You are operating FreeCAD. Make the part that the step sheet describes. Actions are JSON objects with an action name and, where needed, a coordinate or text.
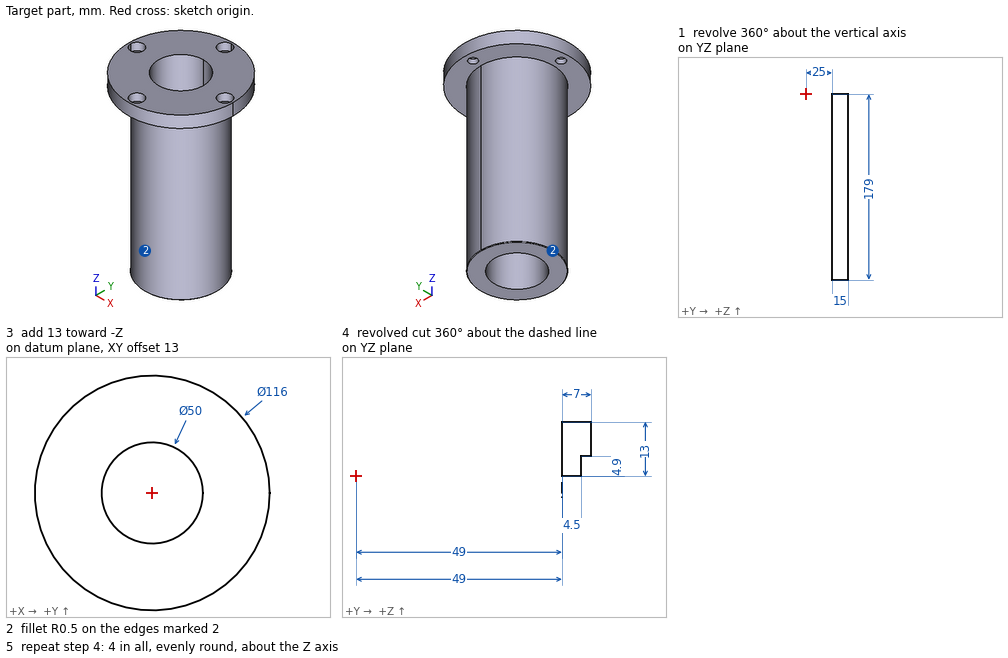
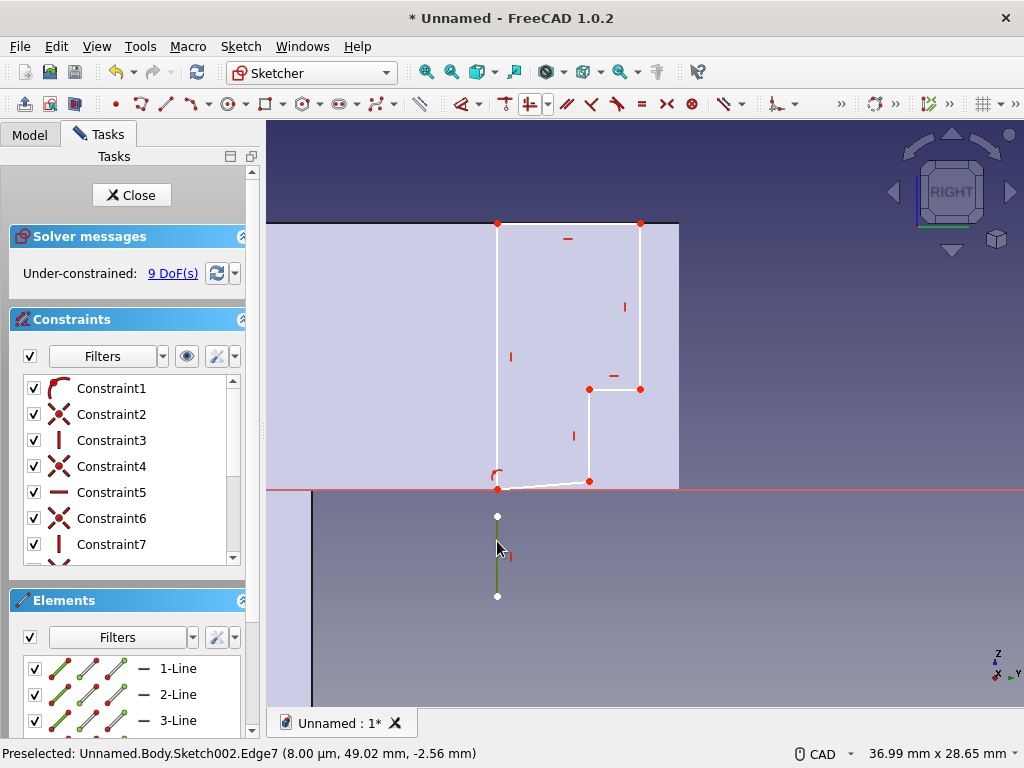
{"action": "left_click", "coordinate": [420, 104]}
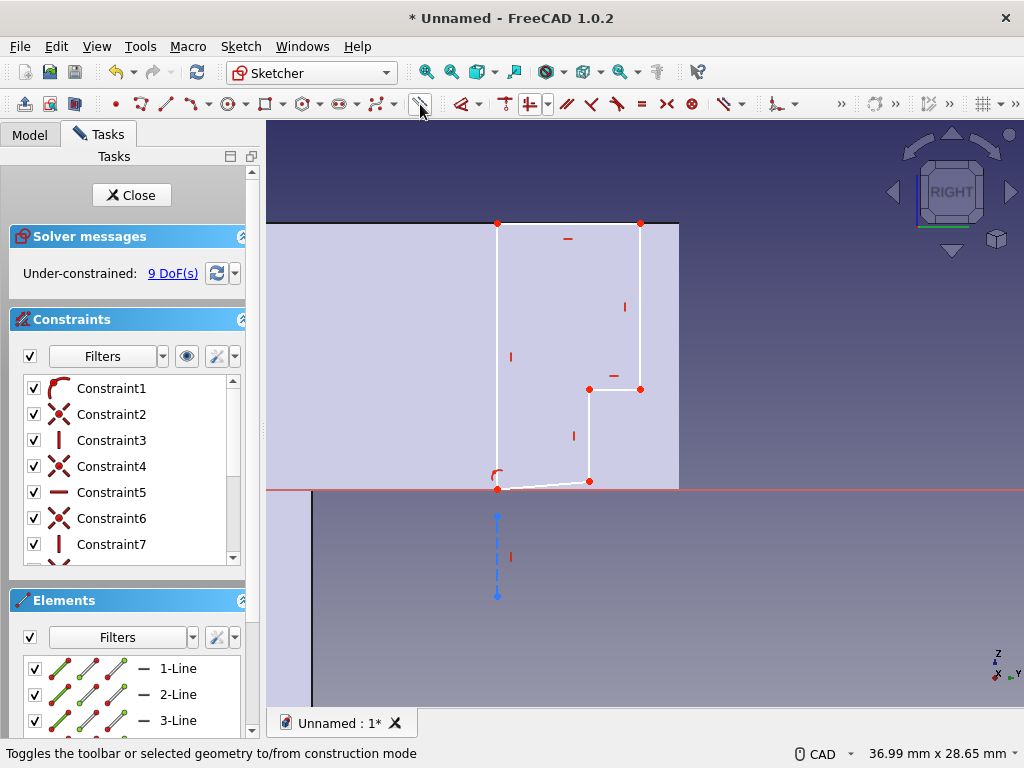
{"action": "left_click", "coordinate": [525, 487]}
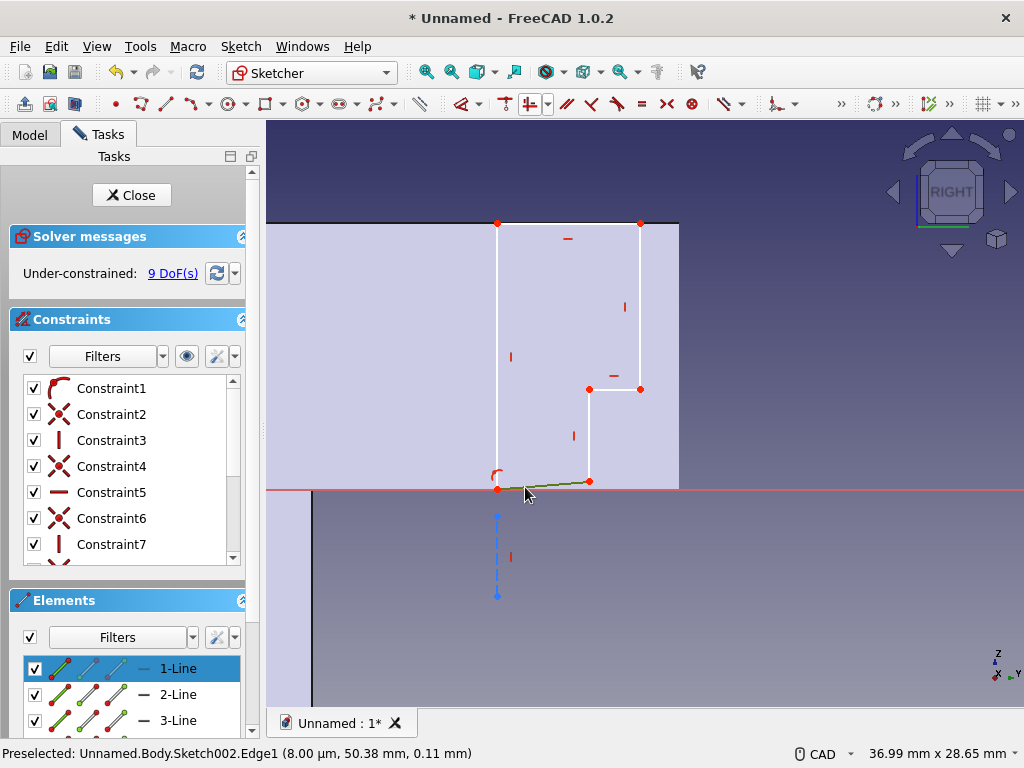
{"action": "left_click", "coordinate": [548, 104]}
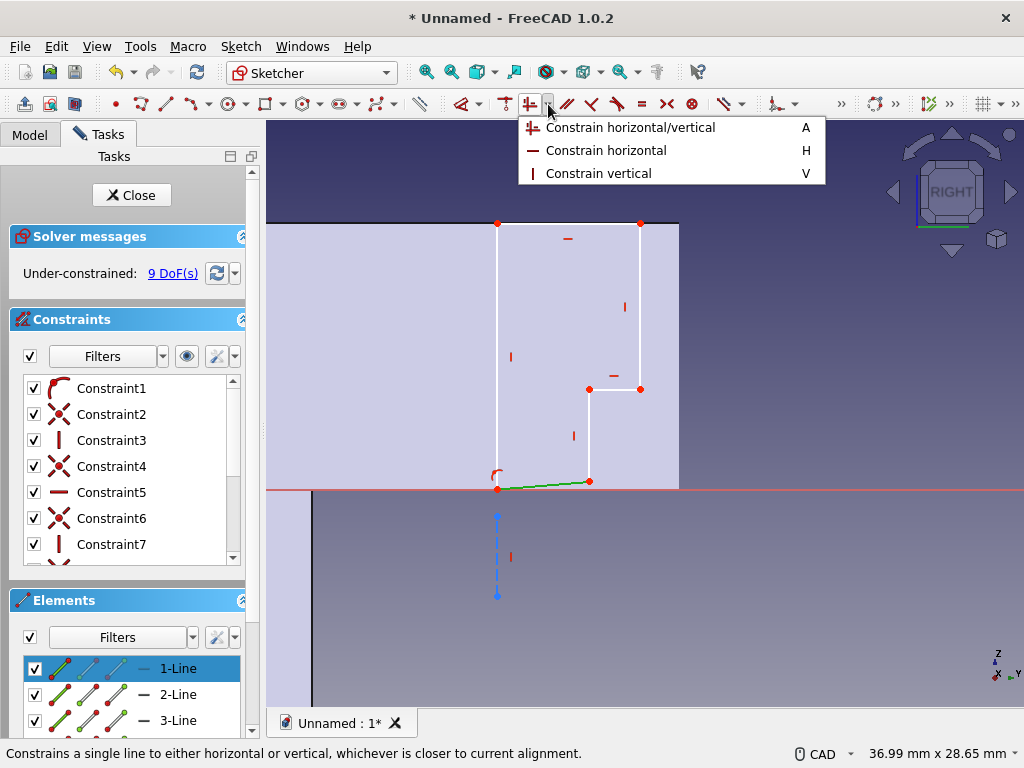
{"action": "left_click", "coordinate": [672, 150]}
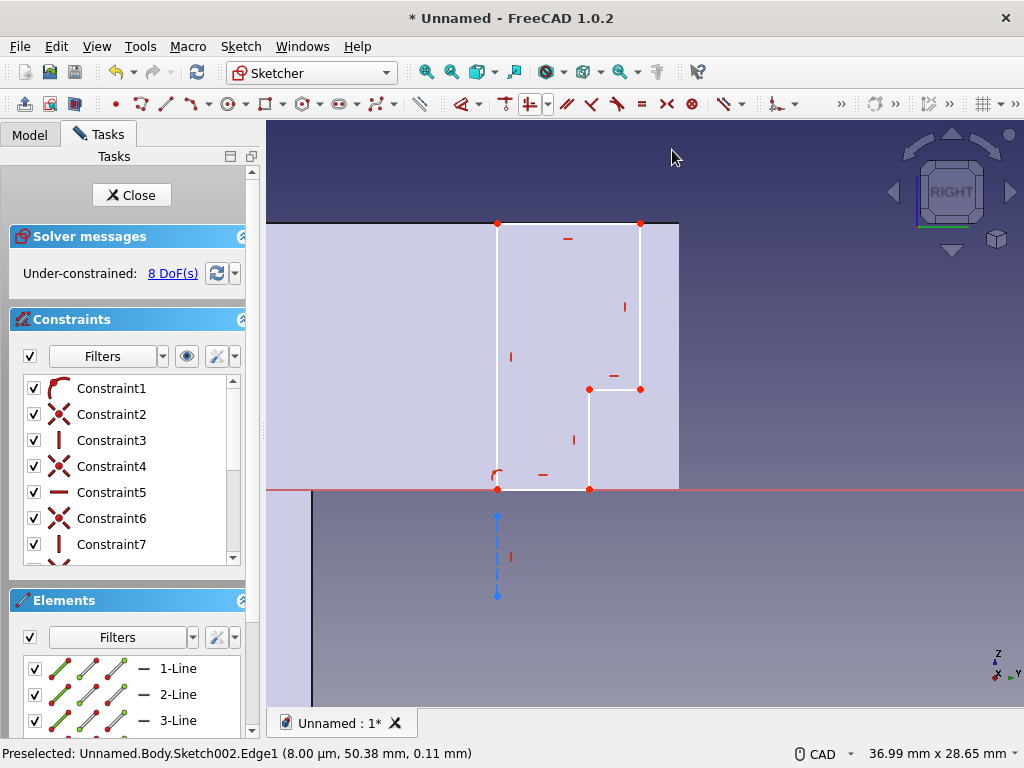
{"action": "left_click", "coordinate": [460, 104]}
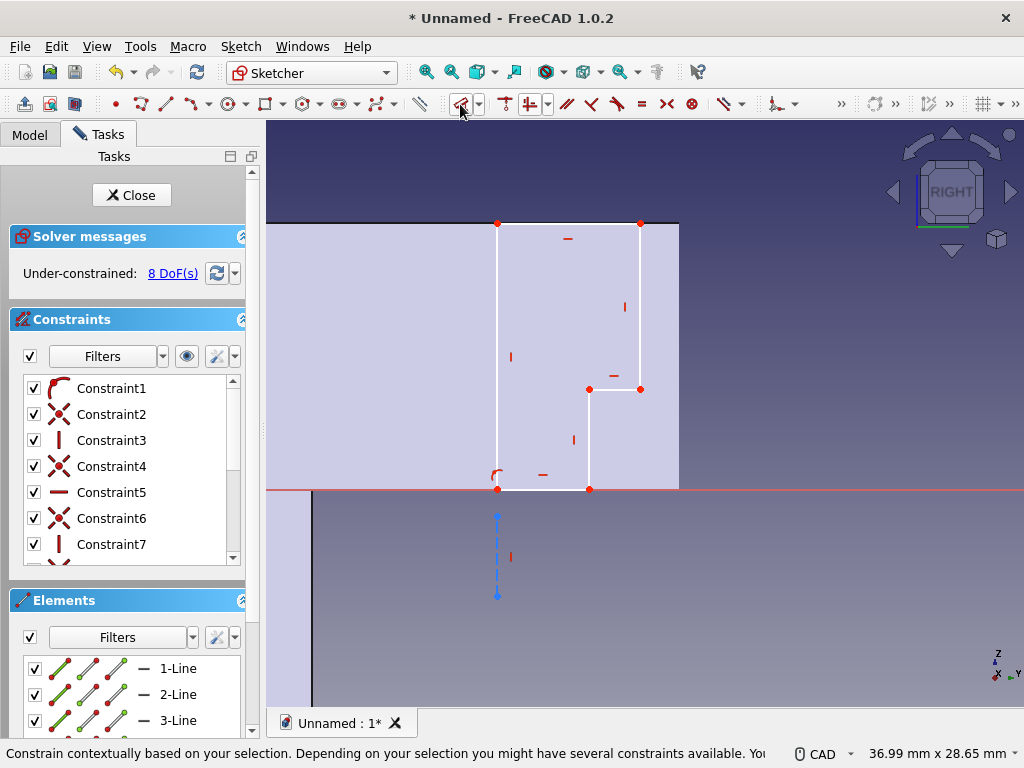
{"action": "left_click", "coordinate": [597, 224]}
{"action": "left_click", "coordinate": [568, 190]}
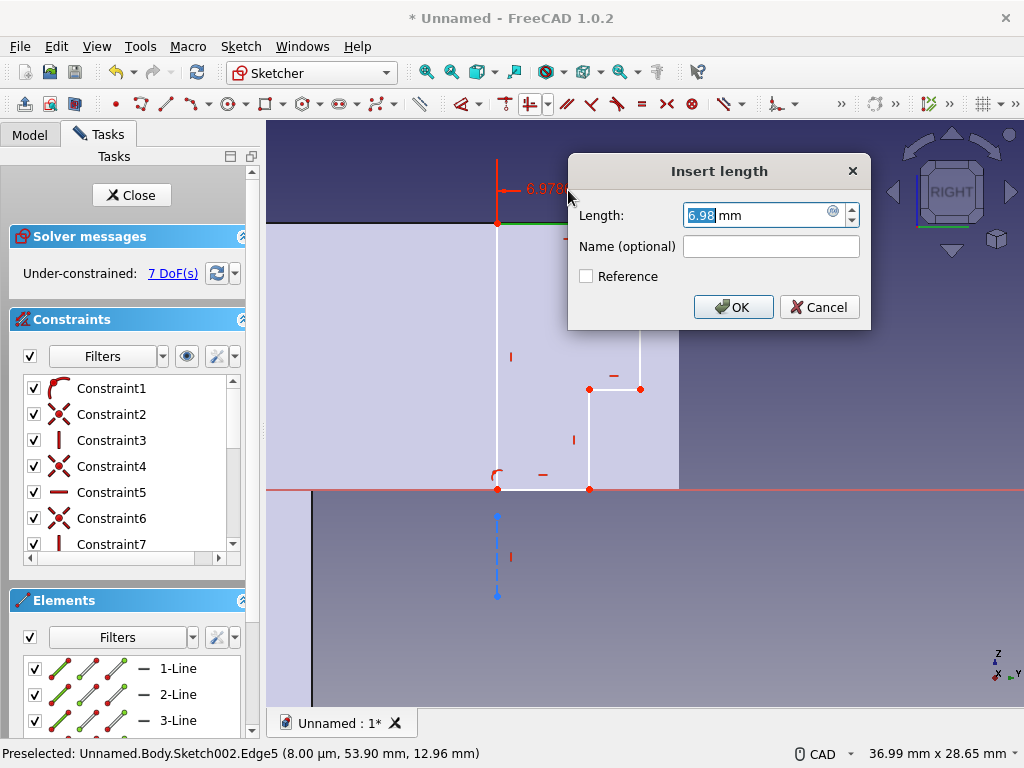
{"action": "type", "text": "7"}
{"action": "key", "text": "Return"}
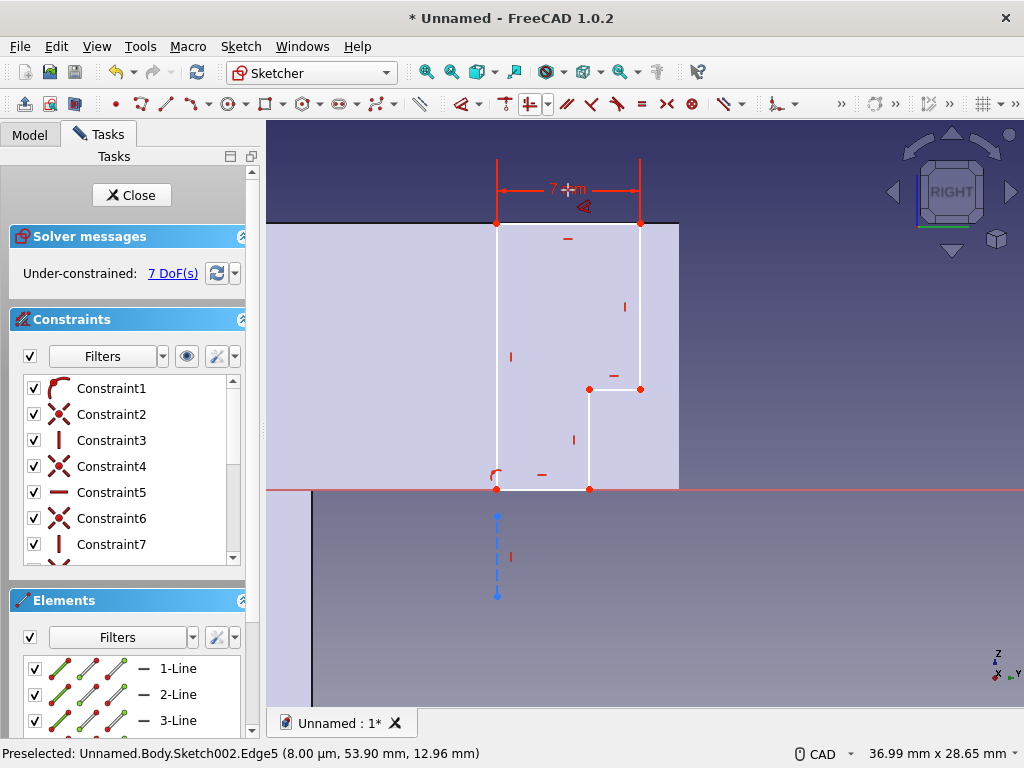
{"action": "left_click", "coordinate": [497, 304]}
{"action": "left_click", "coordinate": [463, 357]}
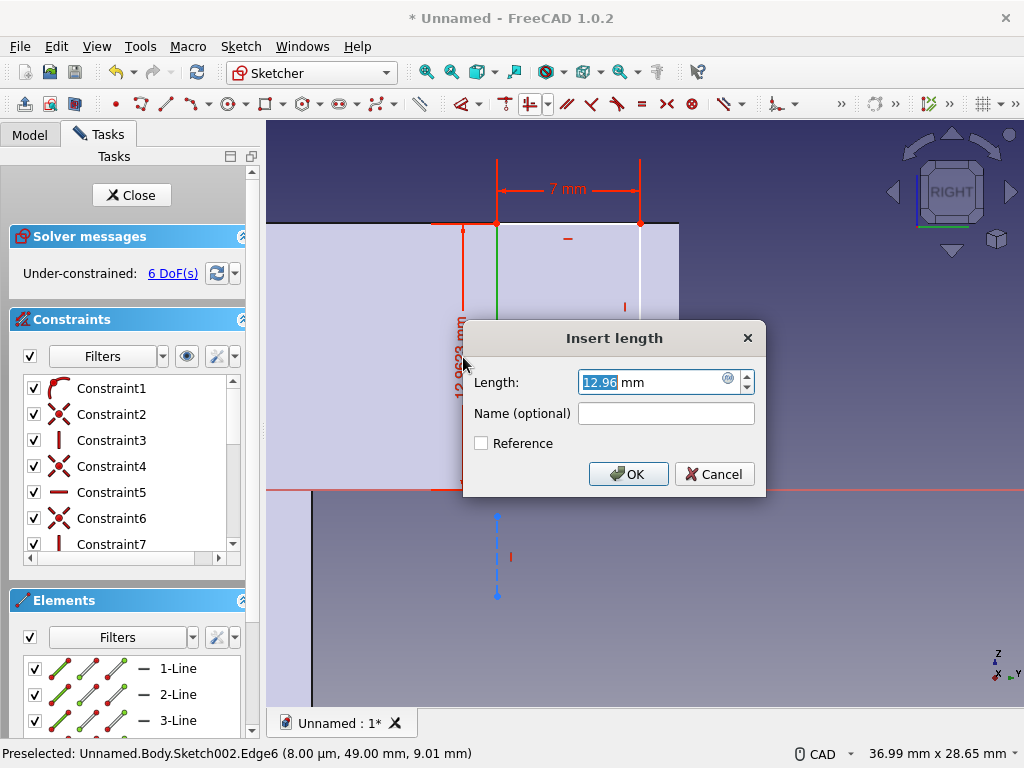
{"action": "type", "text": "13"}
{"action": "key", "text": "Return"}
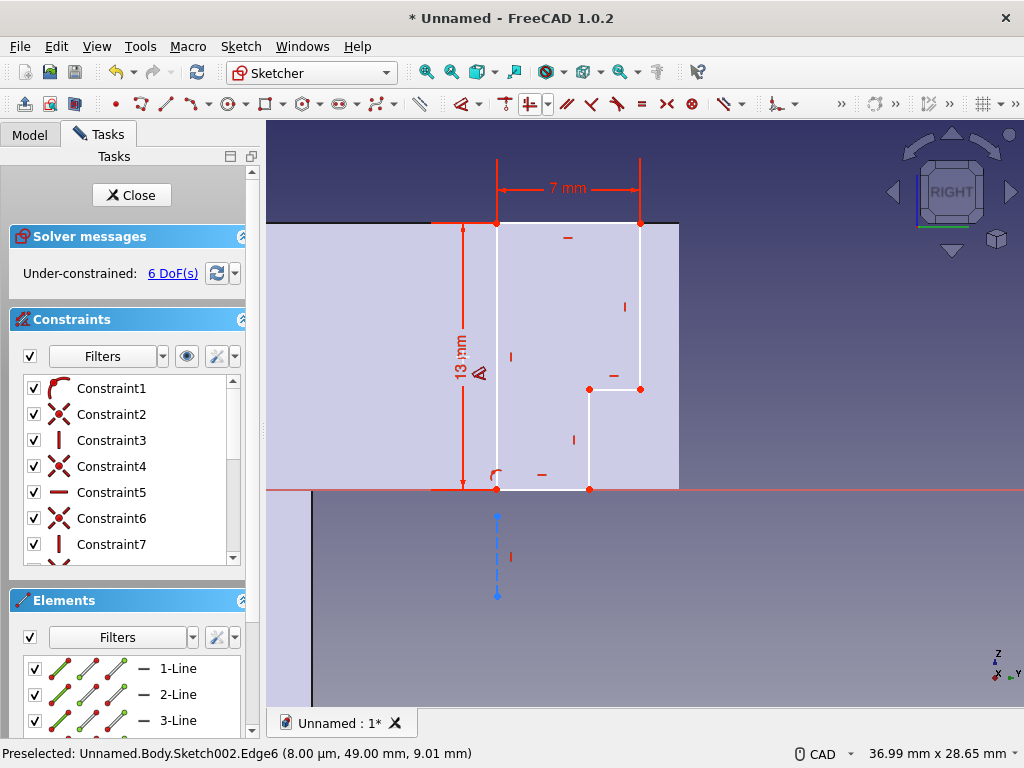
{"action": "left_click", "coordinate": [524, 490]}
{"action": "left_click", "coordinate": [543, 524]}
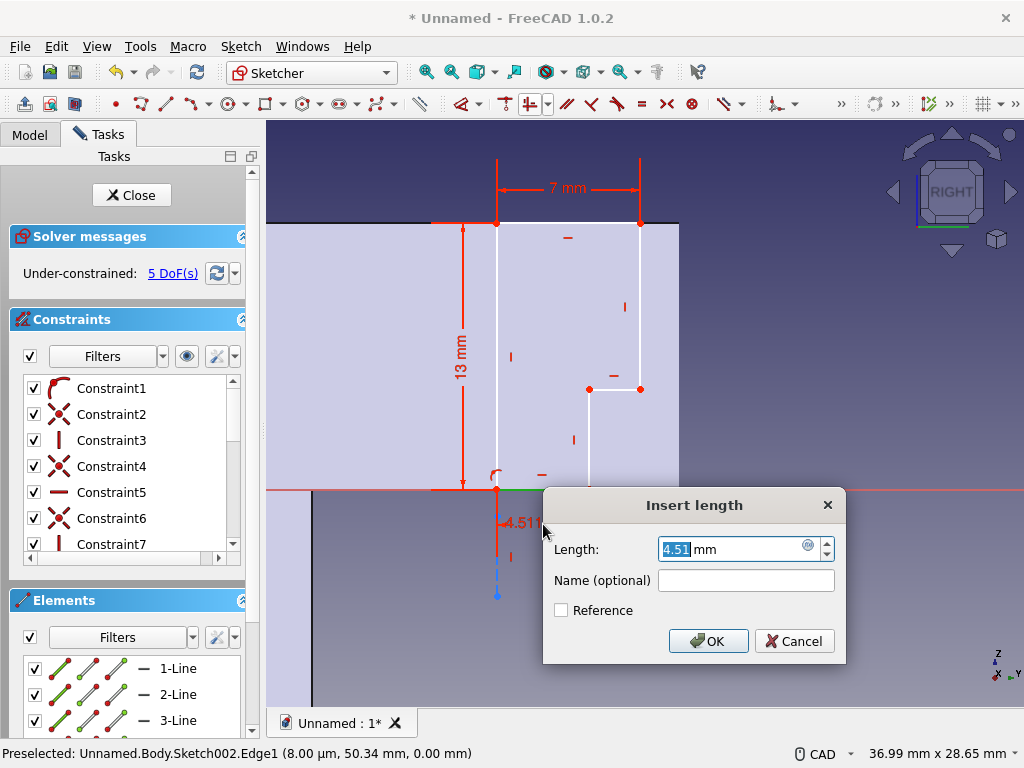
{"action": "type", "text": "4.5"}
{"action": "key", "text": "Return"}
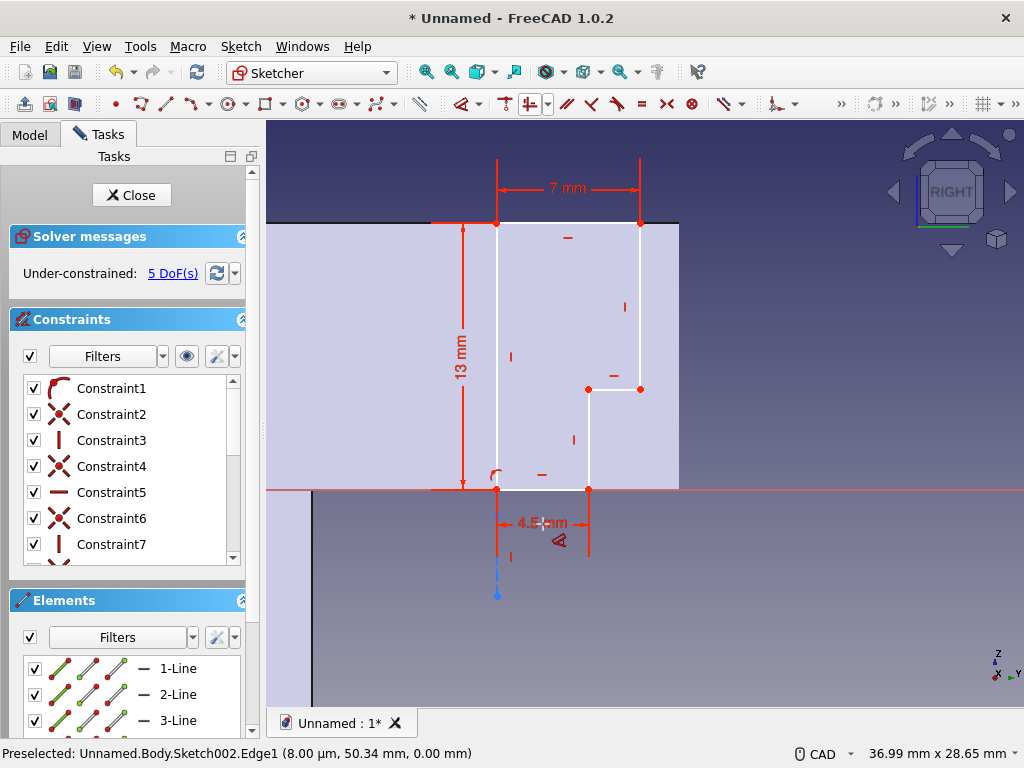
{"action": "left_click", "coordinate": [589, 460]}
{"action": "left_click", "coordinate": [623, 440]}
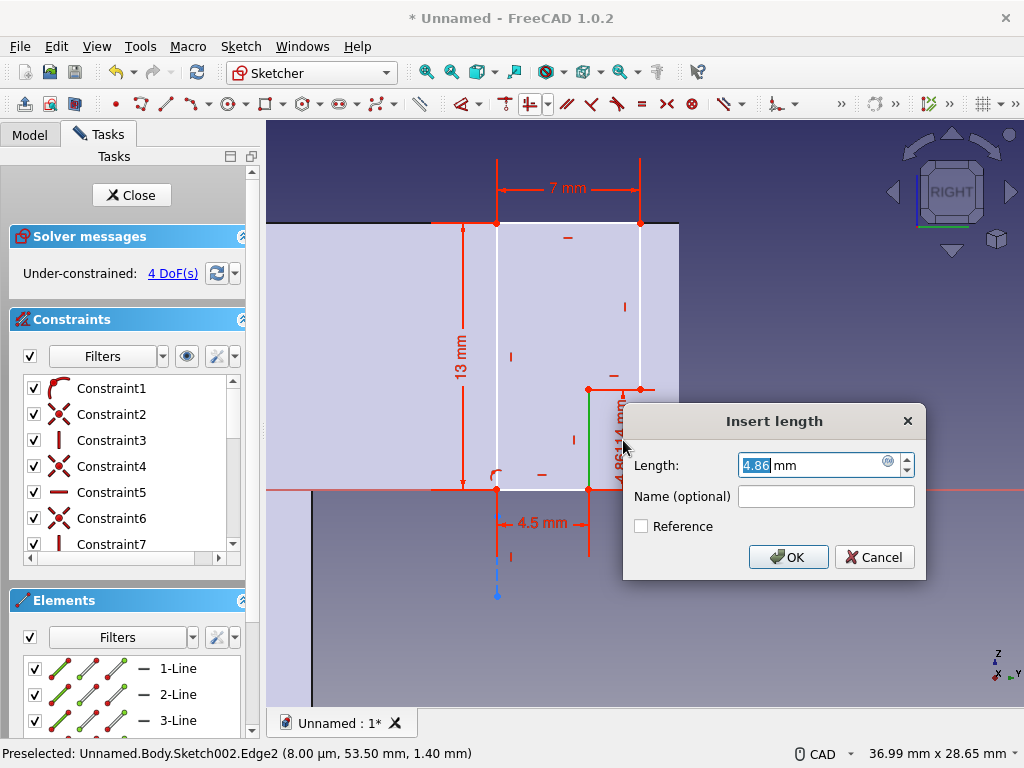
{"action": "type", "text": "4.9"}
{"action": "key", "text": "Return"}